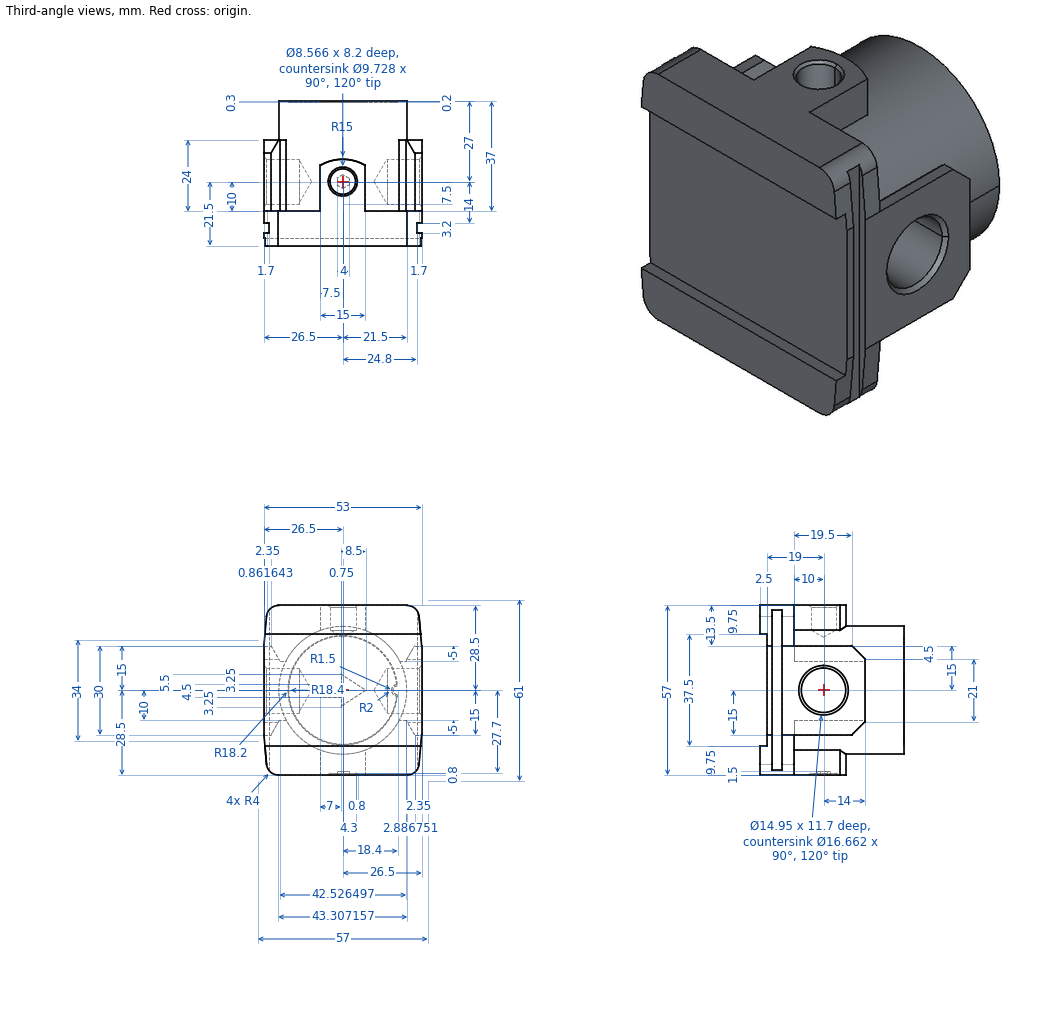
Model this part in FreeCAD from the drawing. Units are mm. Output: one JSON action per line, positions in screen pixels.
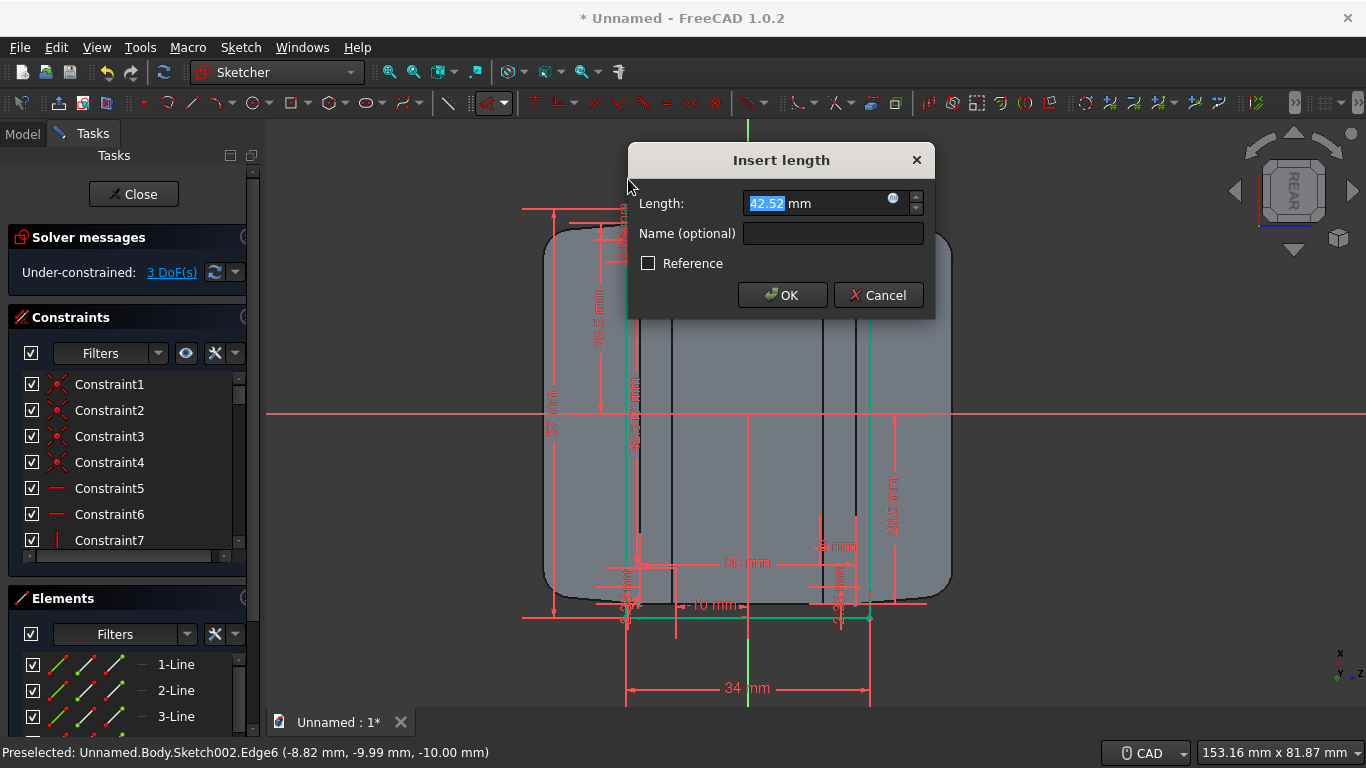
{"action": "type", "text": "42.526497"}
{"action": "key", "text": "Return"}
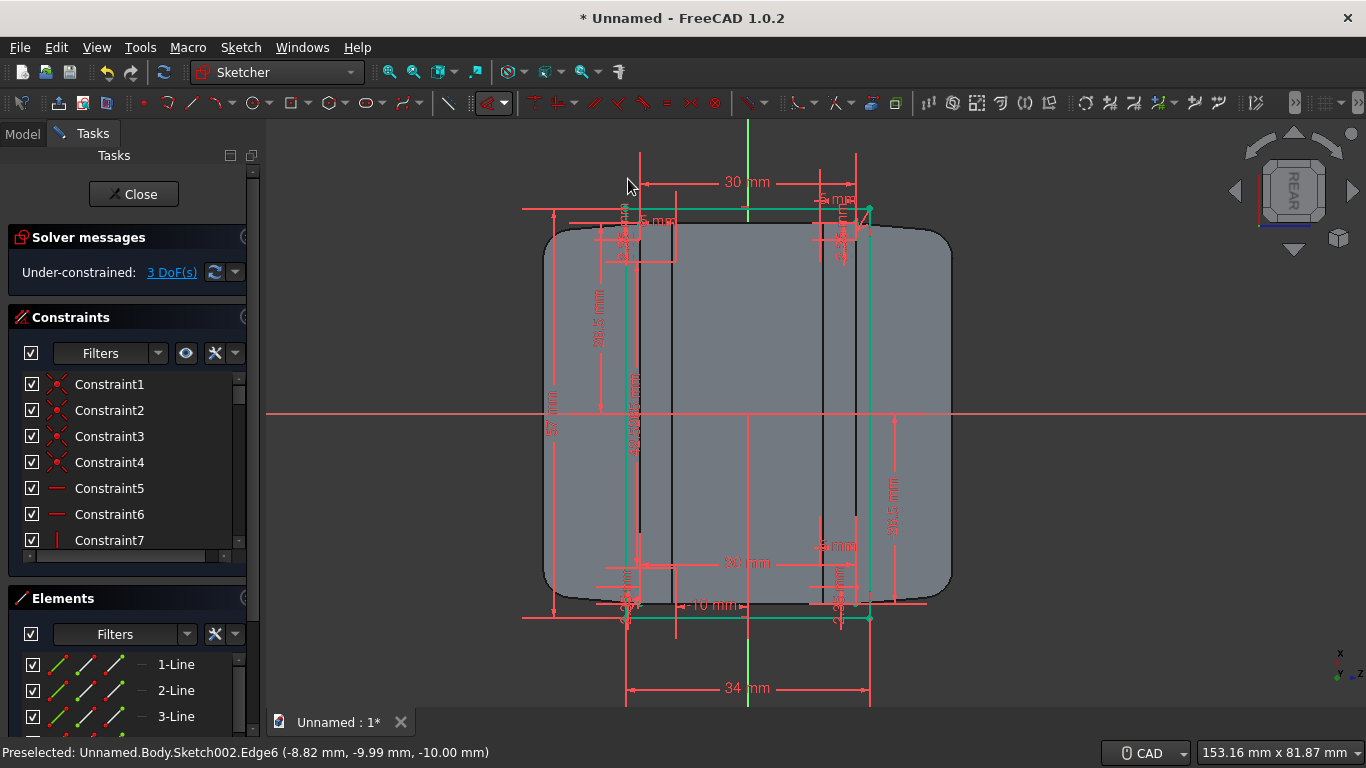
{"action": "left_click", "coordinate": [820, 353]}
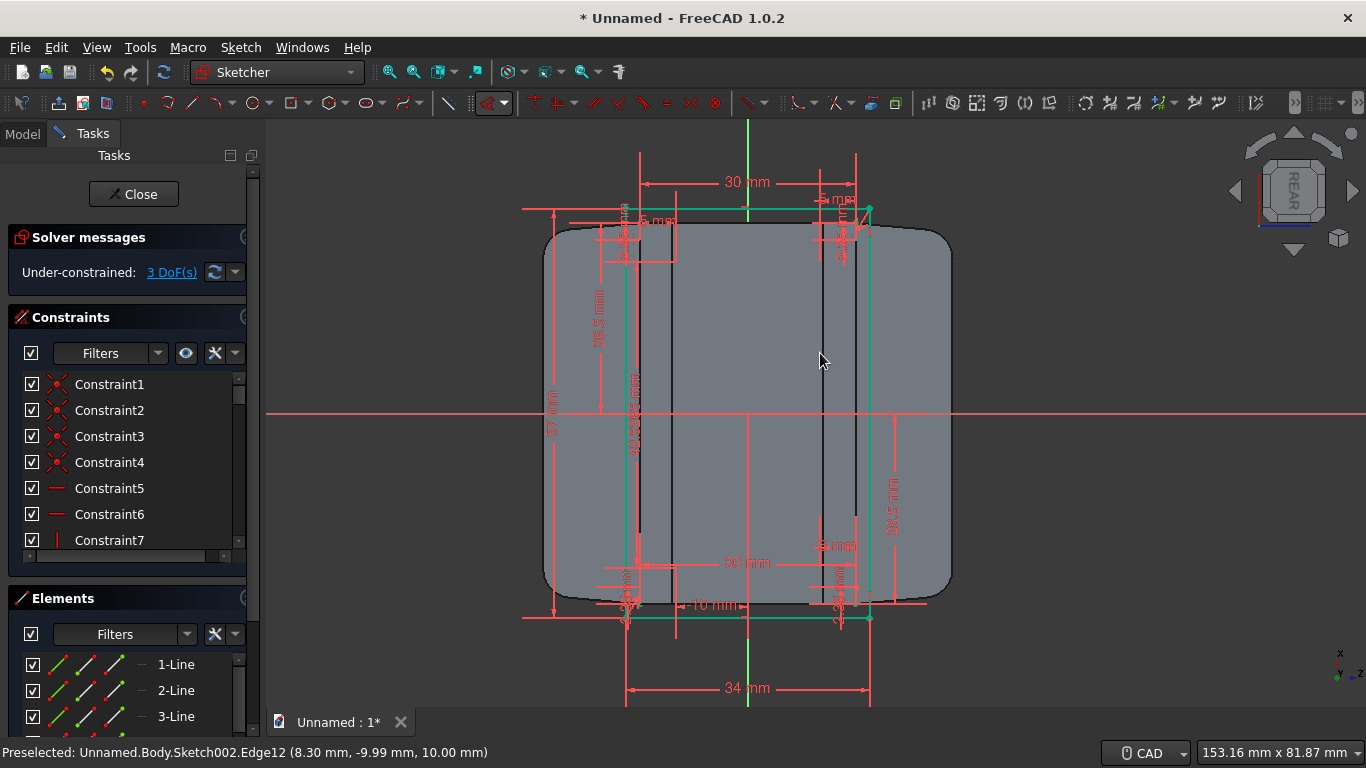
{"action": "left_click", "coordinate": [506, 104]}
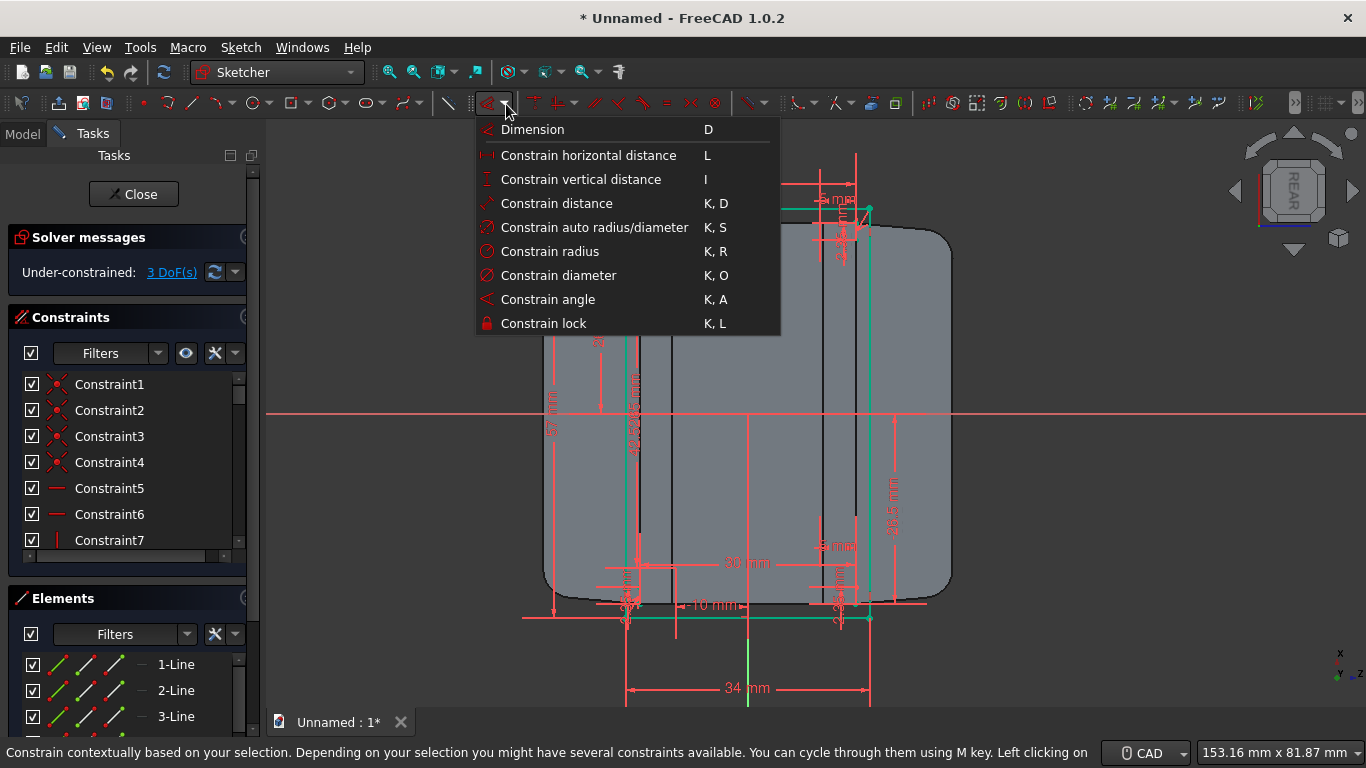
{"action": "left_click", "coordinate": [628, 179]}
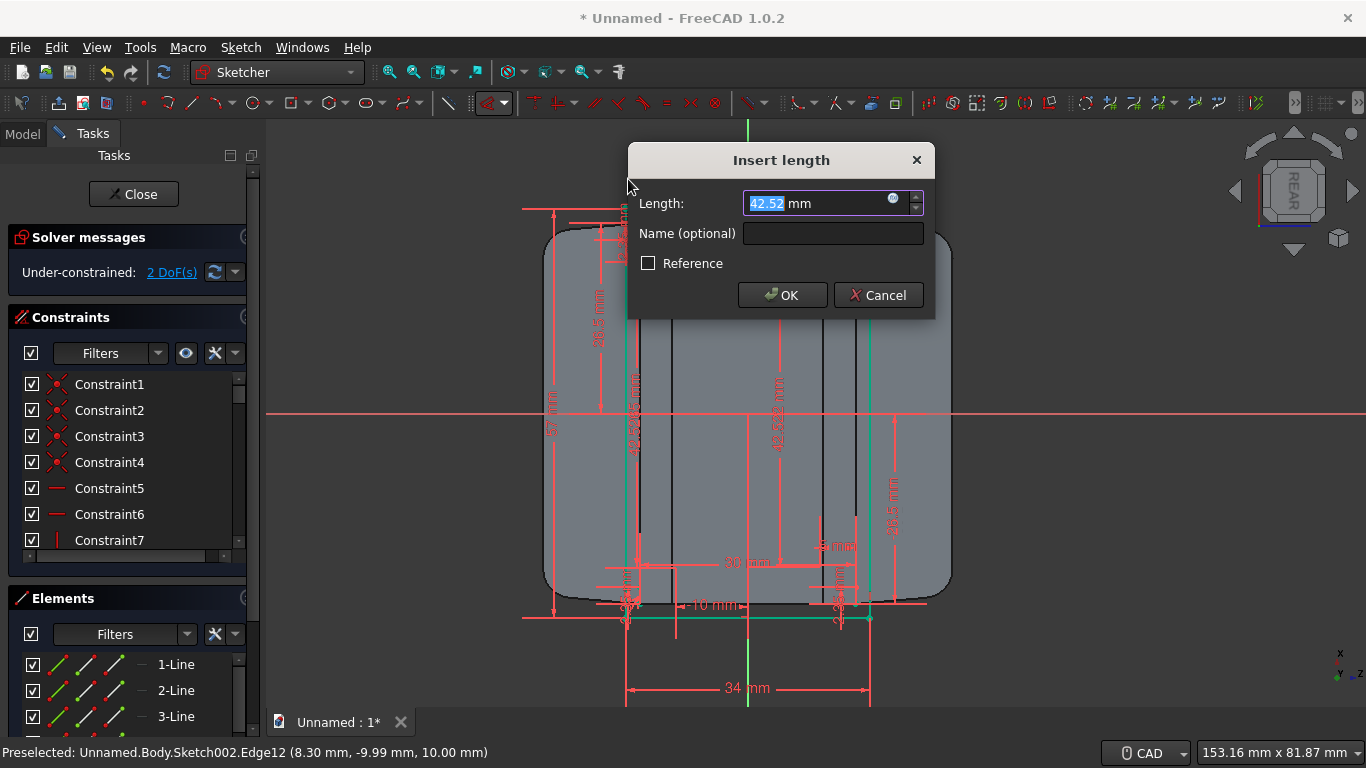
{"action": "type", "text": "42.526497"}
{"action": "key", "text": "Return"}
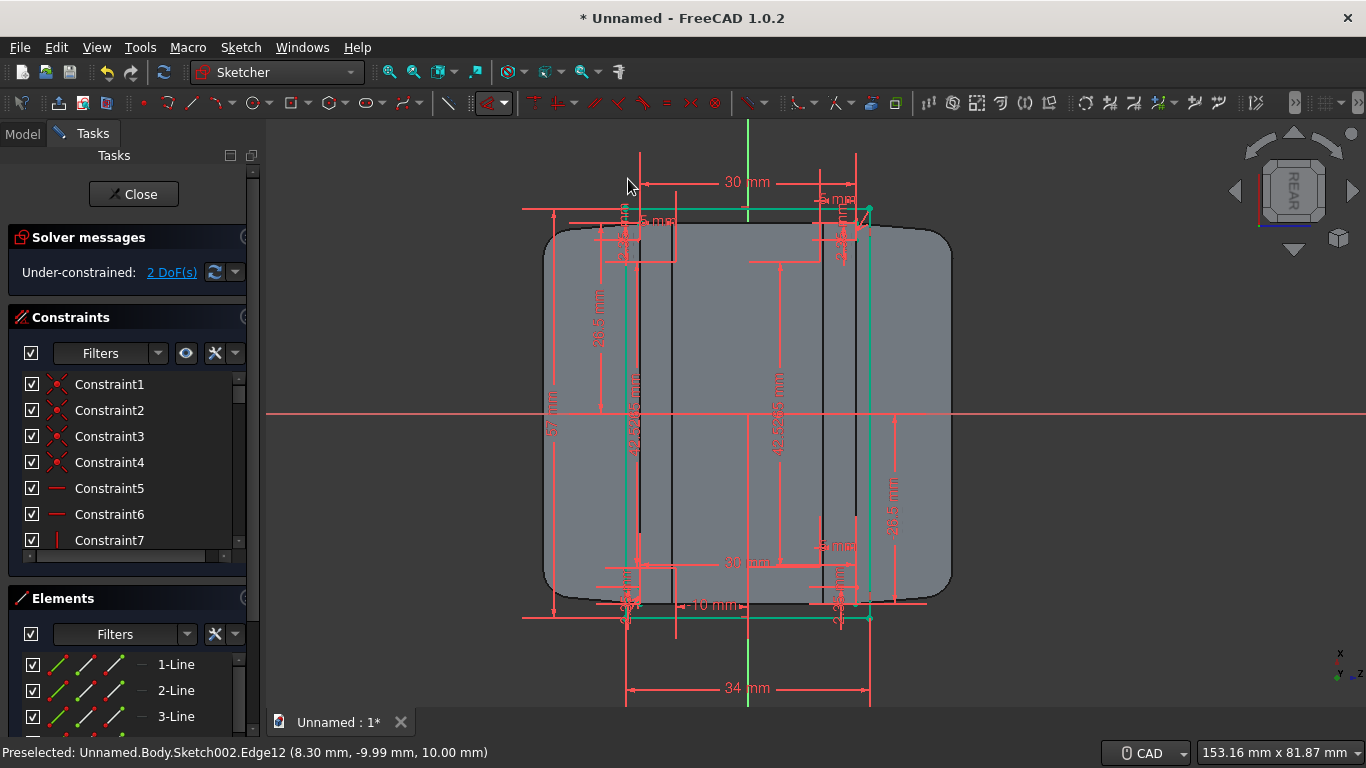
{"action": "scroll", "coordinate": [665, 256], "scroll_direction": "up", "scroll_amount": 4}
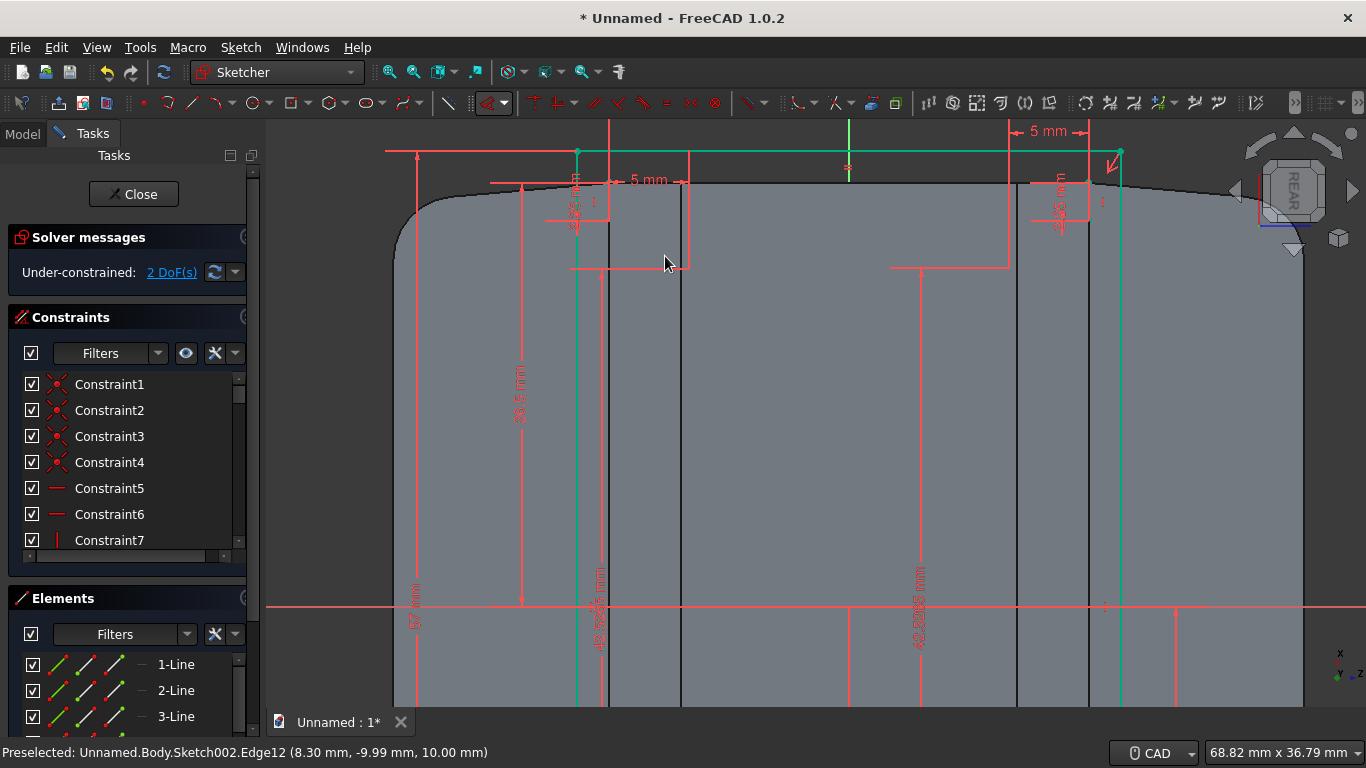
{"action": "left_click", "coordinate": [665, 255]}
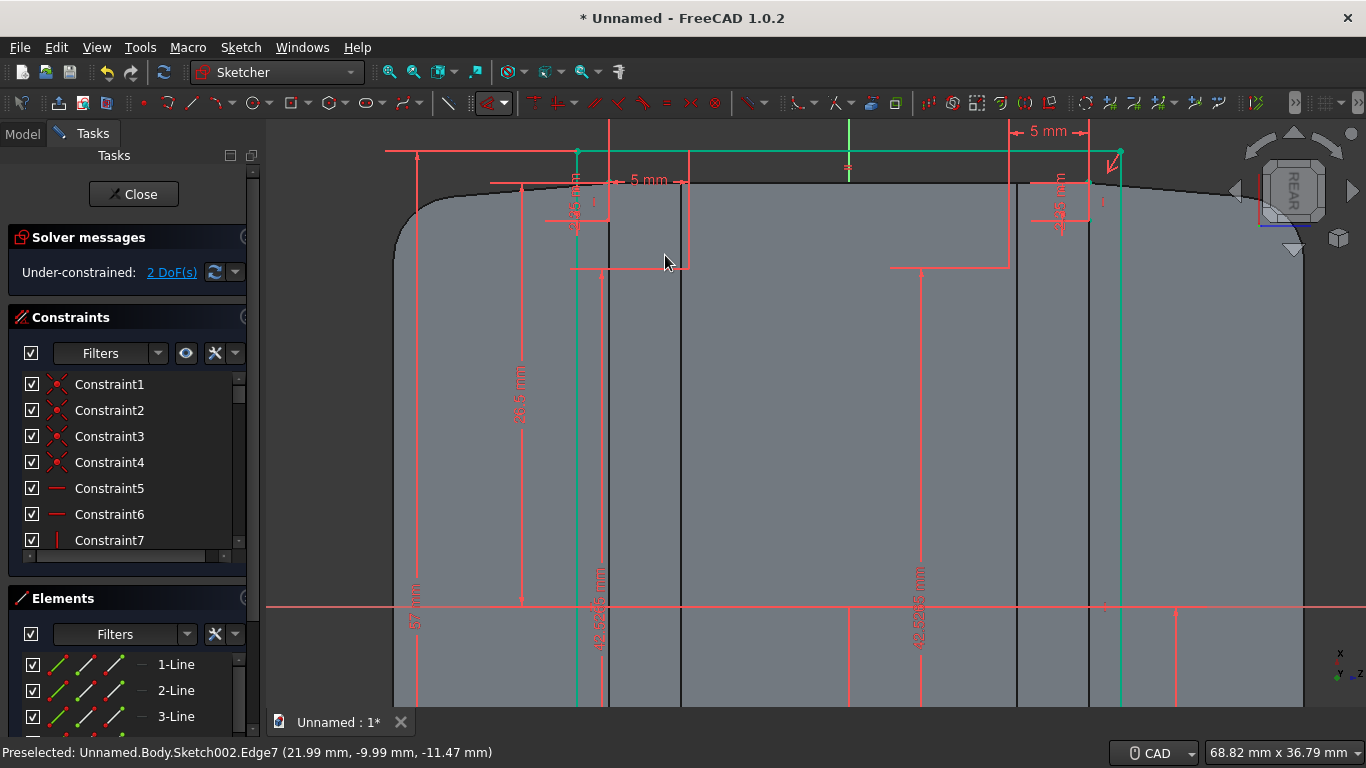
{"action": "left_click", "coordinate": [506, 104]}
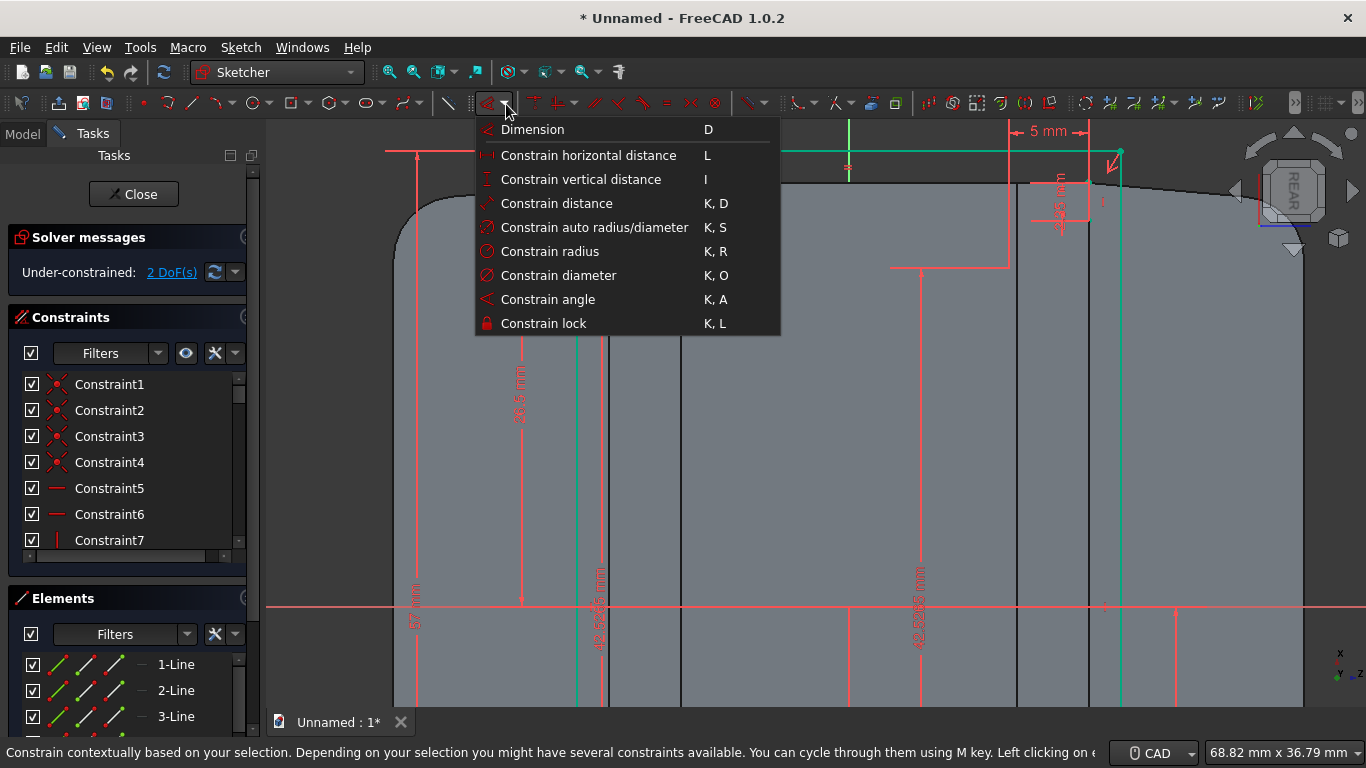
{"action": "left_click", "coordinate": [628, 179]}